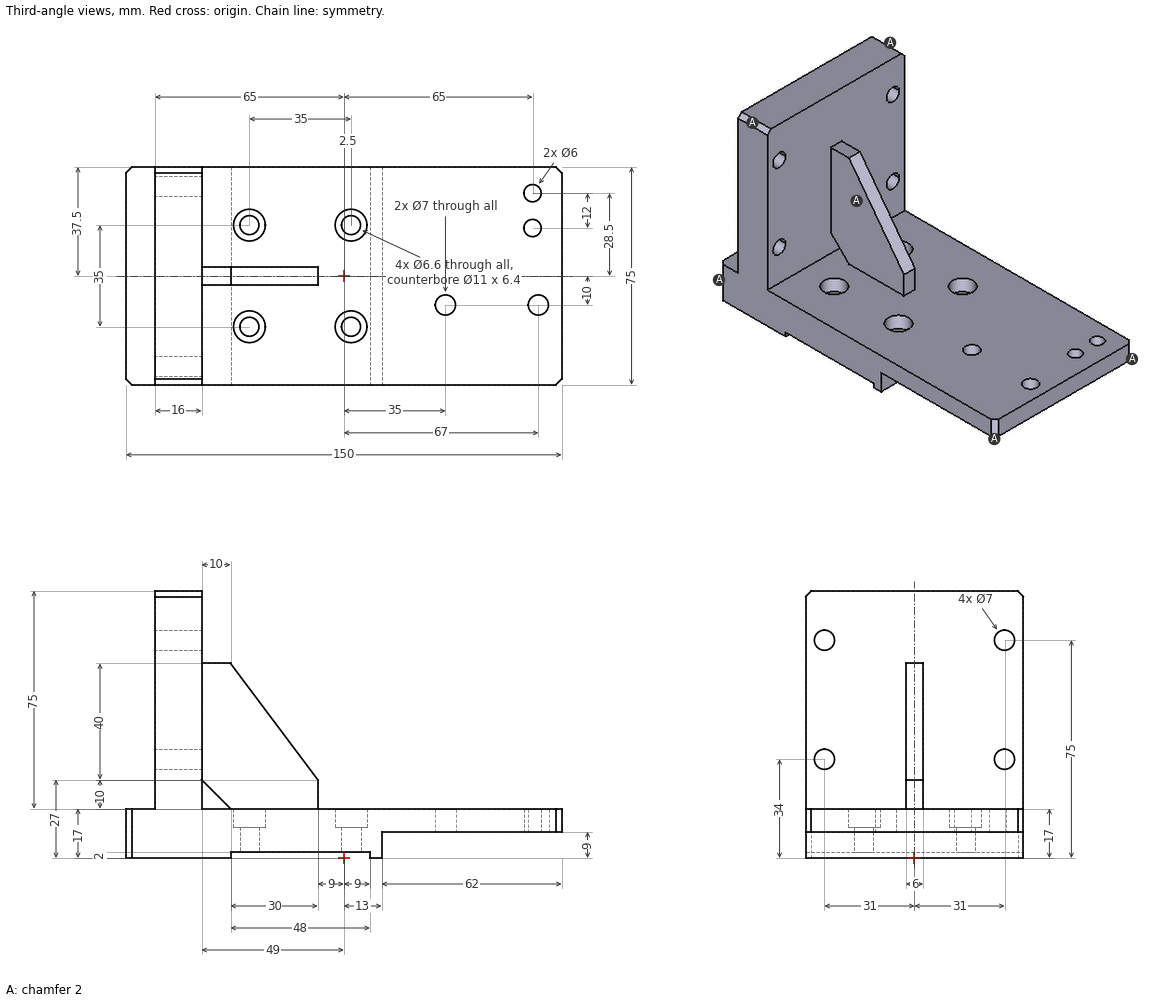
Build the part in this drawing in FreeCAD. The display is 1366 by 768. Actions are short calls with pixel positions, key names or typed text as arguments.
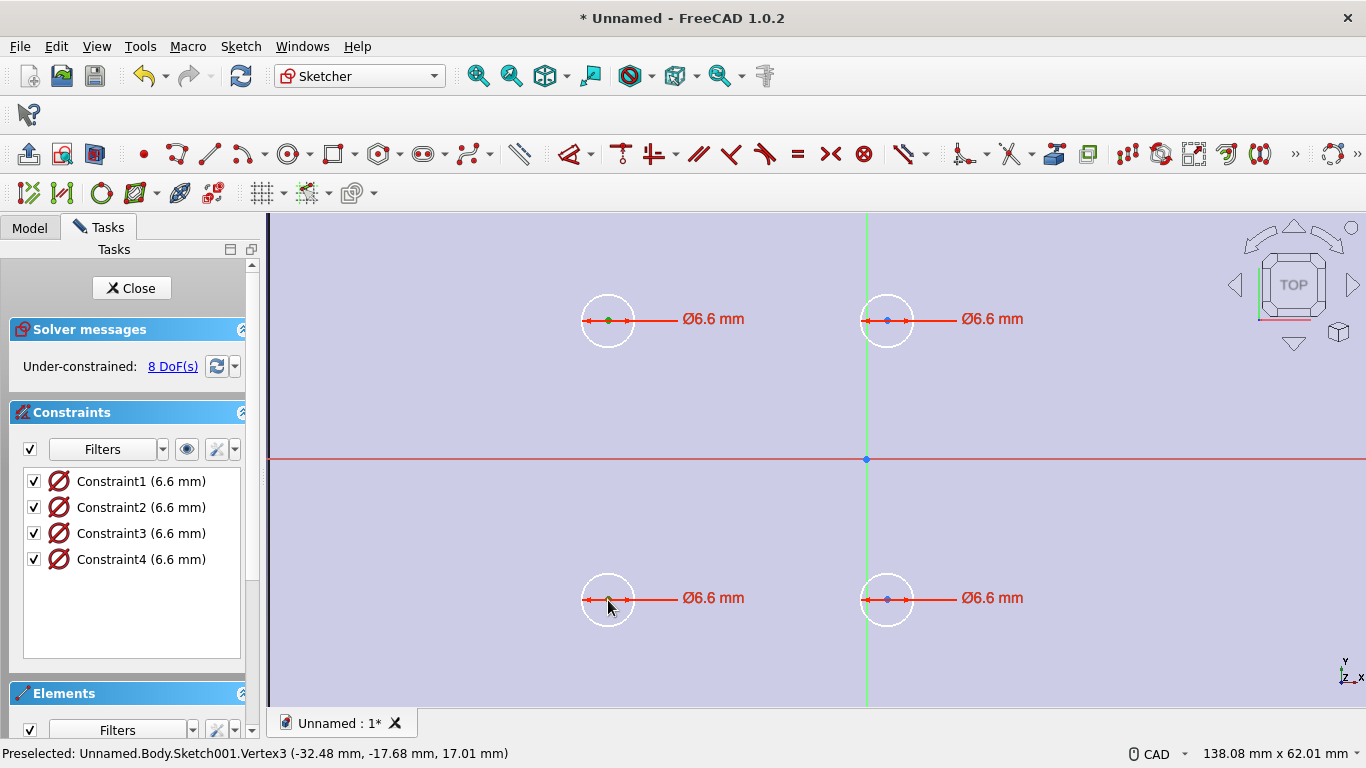
click(359, 459)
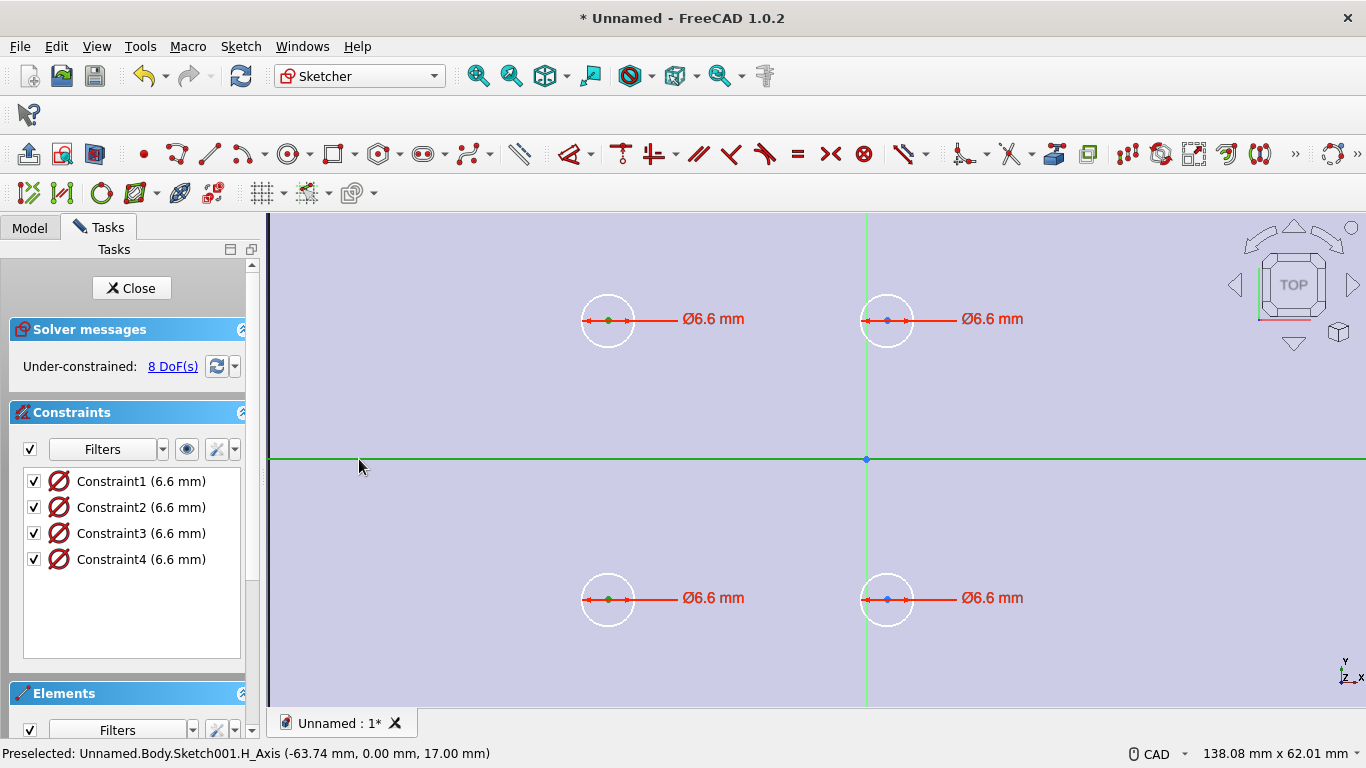
click(831, 154)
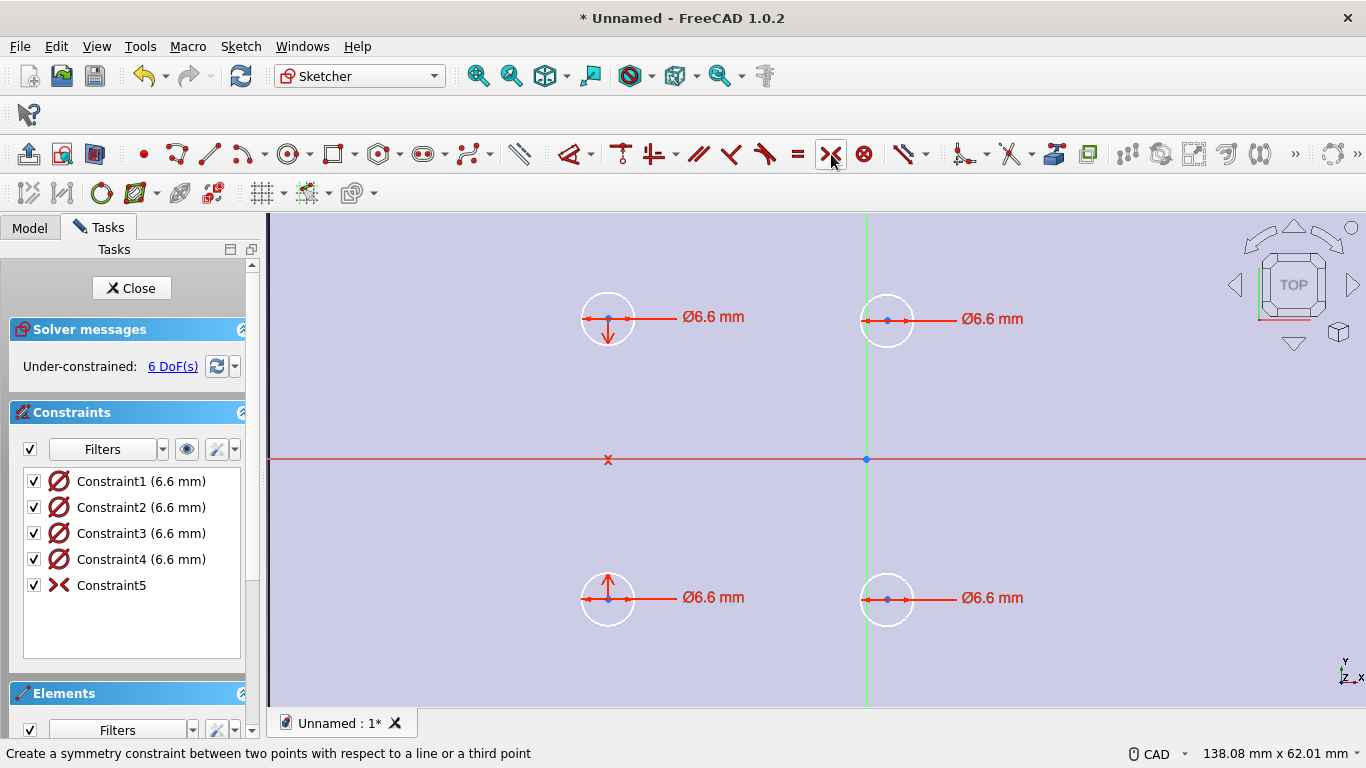
click(887, 321)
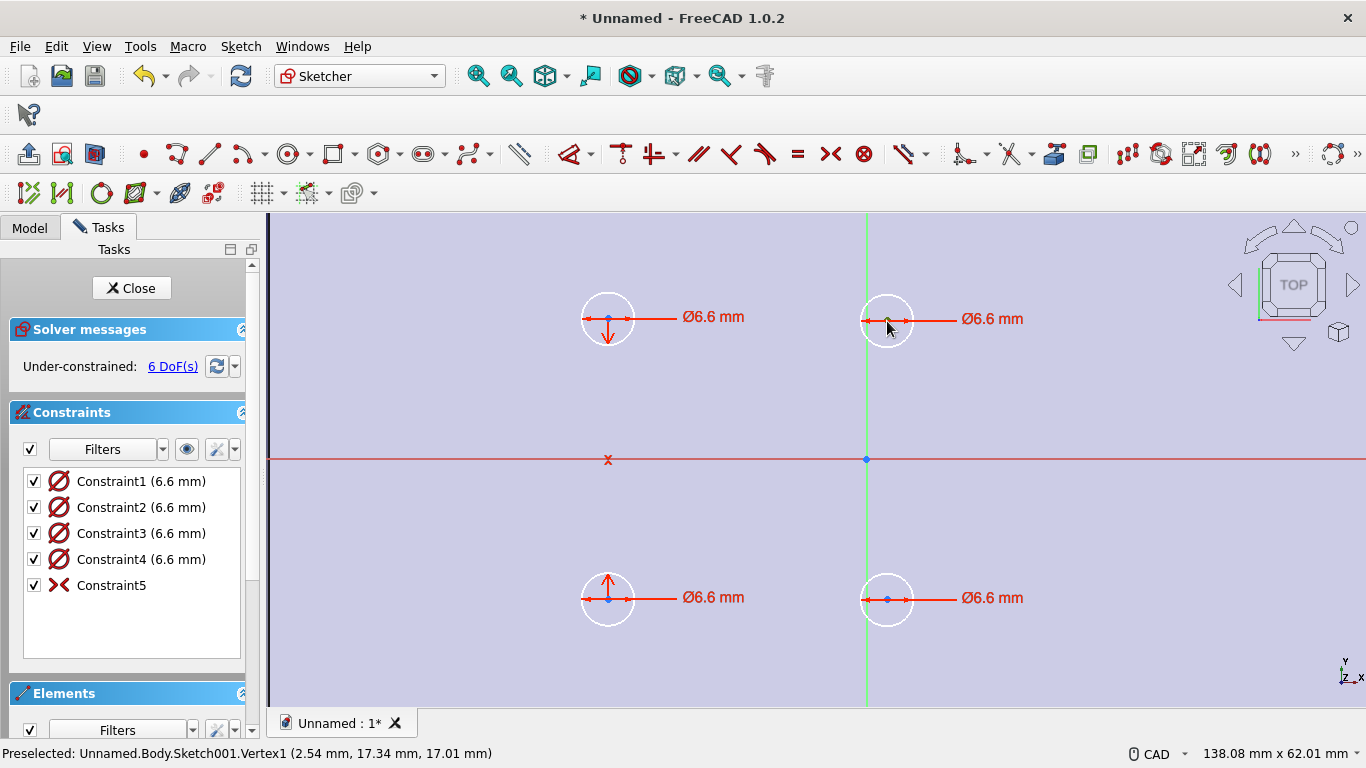
click(887, 600)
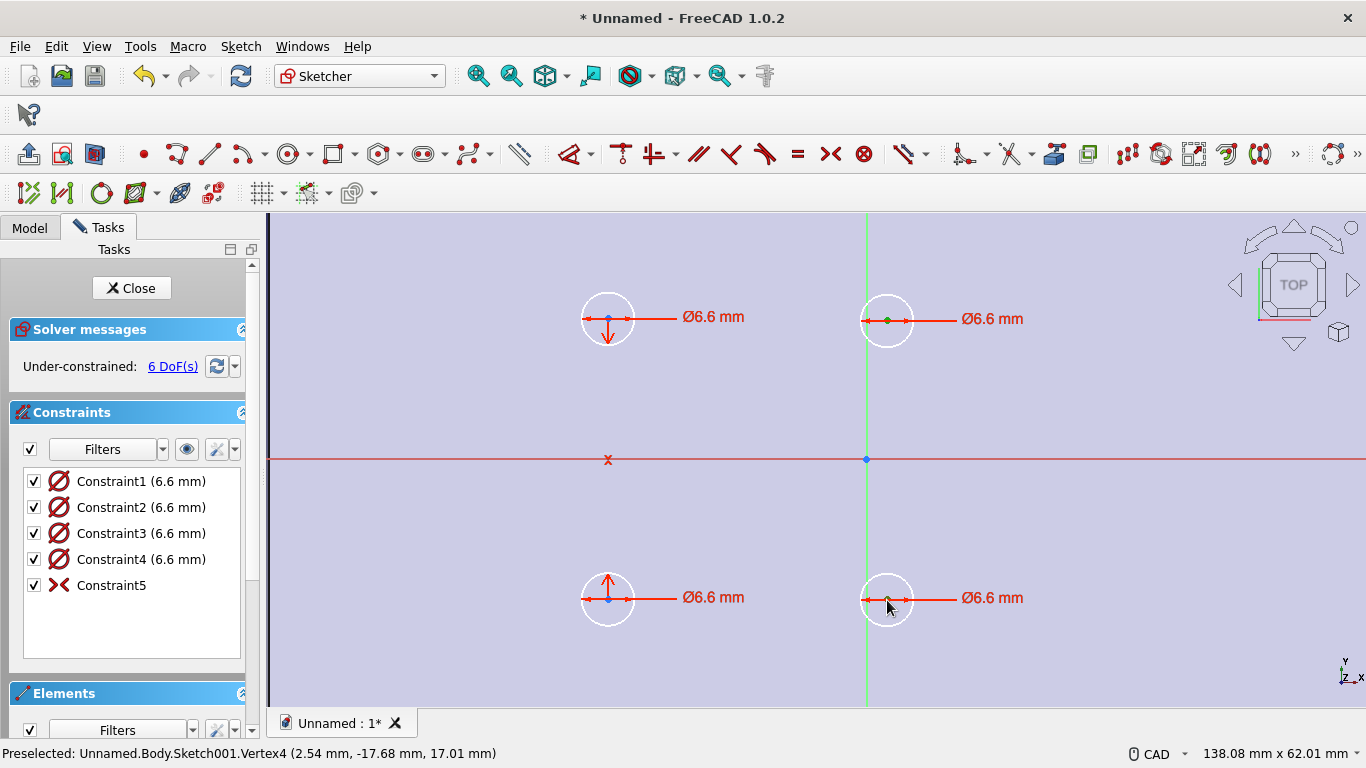
click(359, 459)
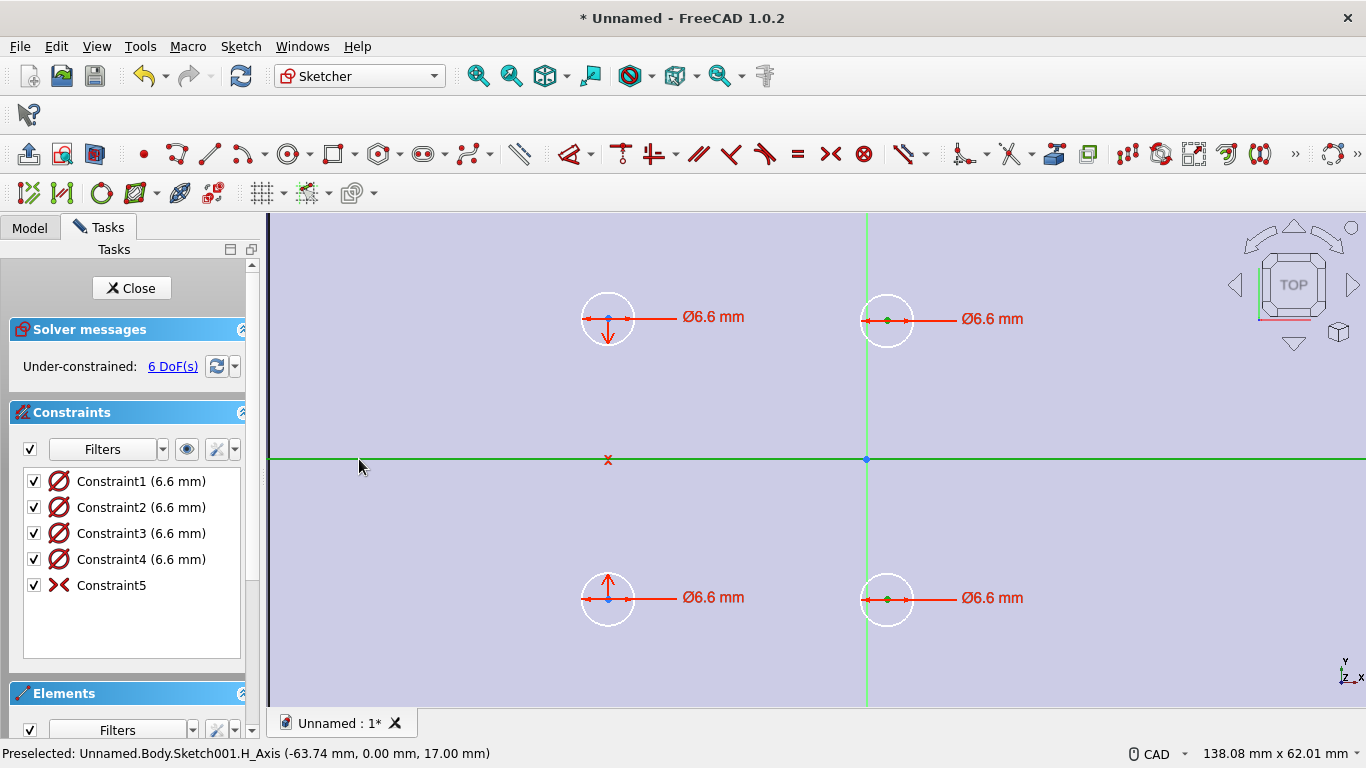
click(831, 154)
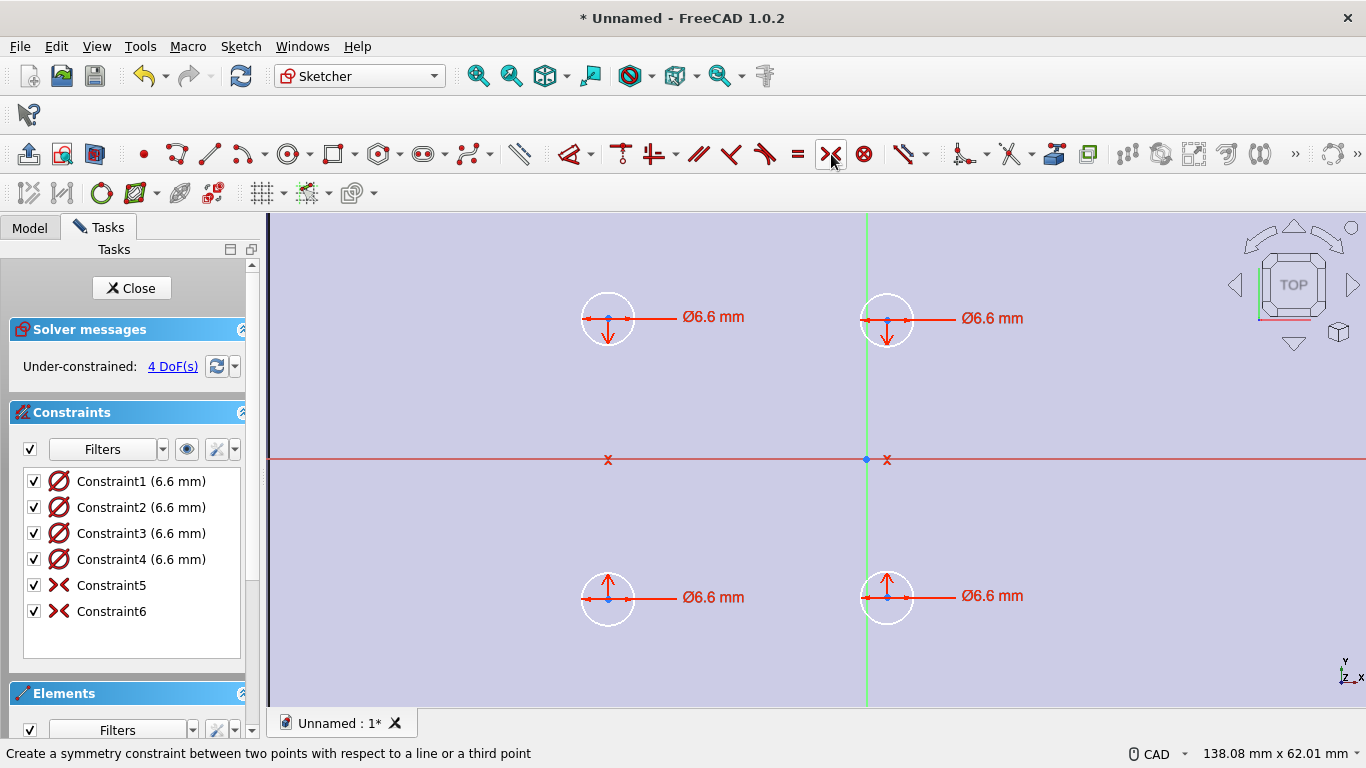
click(568, 154)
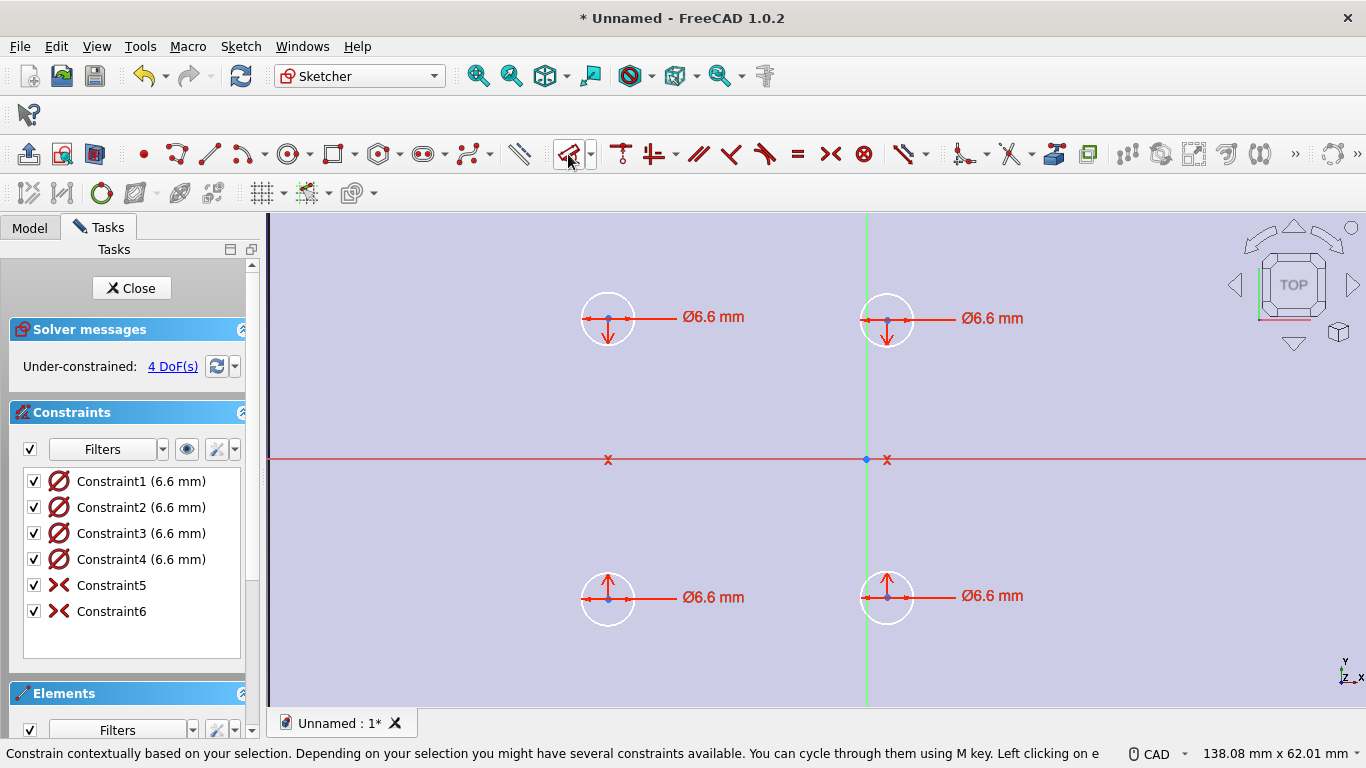
scroll(887, 320, up, 4)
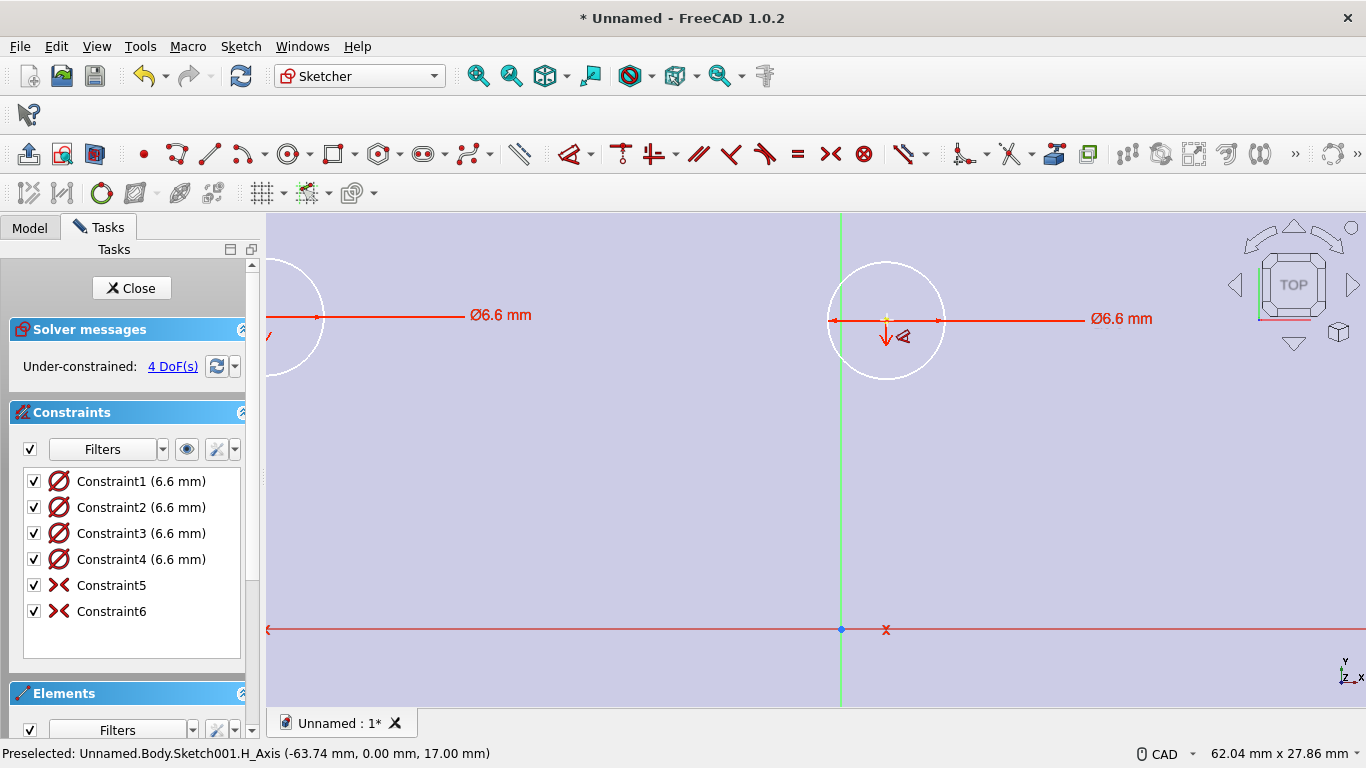
click(886, 321)
click(864, 287)